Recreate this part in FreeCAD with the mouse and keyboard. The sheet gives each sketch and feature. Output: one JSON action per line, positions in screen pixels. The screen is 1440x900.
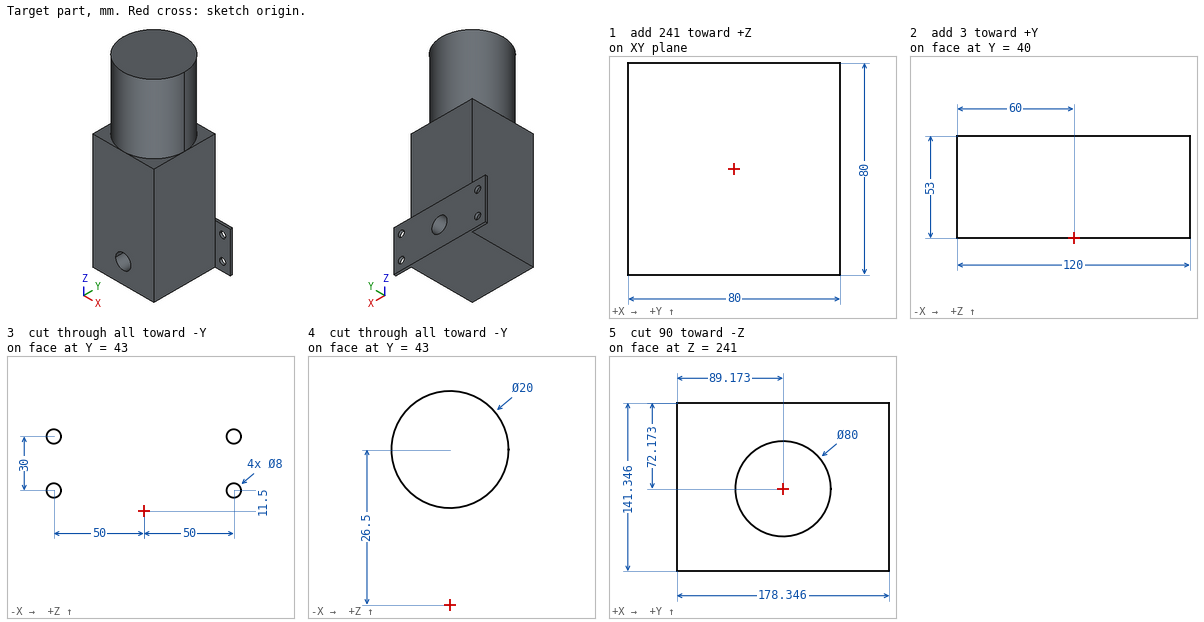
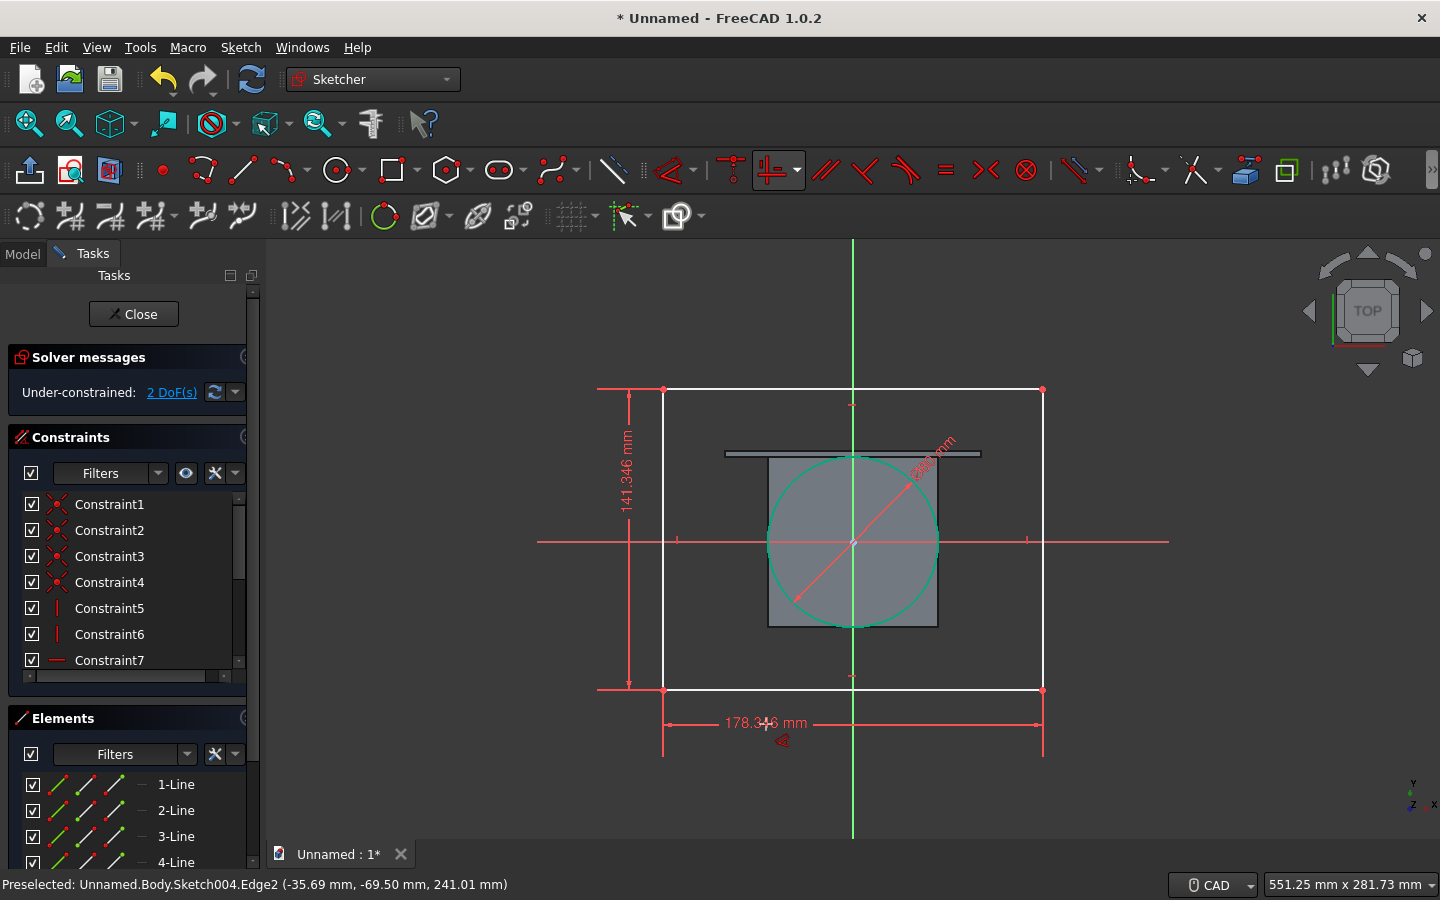
{"action": "left_click", "coordinate": [663, 389]}
{"action": "left_click", "coordinate": [758, 355]}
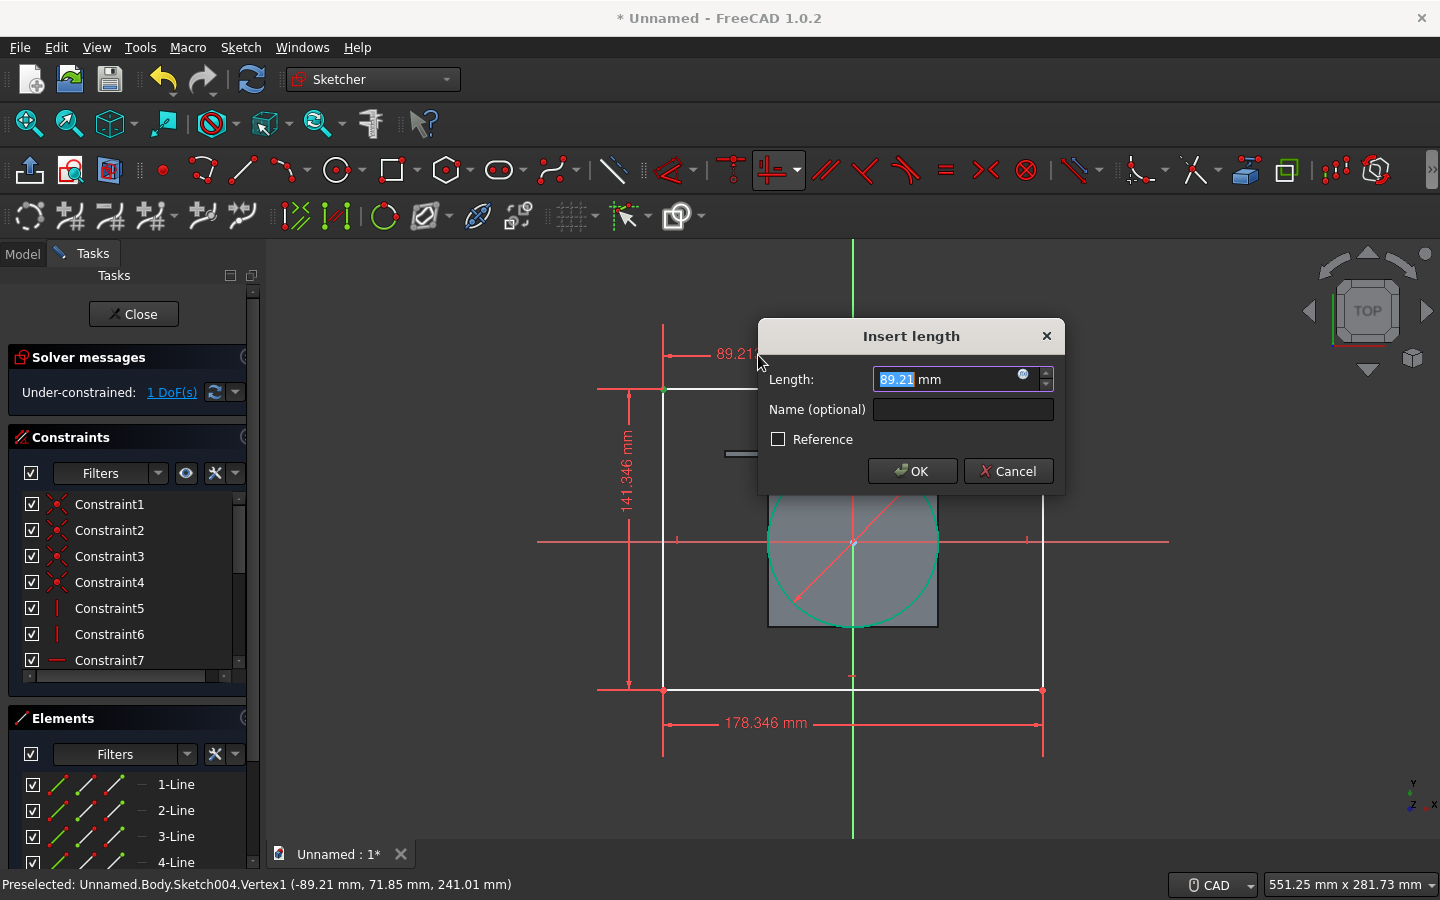
{"action": "type", "text": "89.173"}
{"action": "key", "text": "Return"}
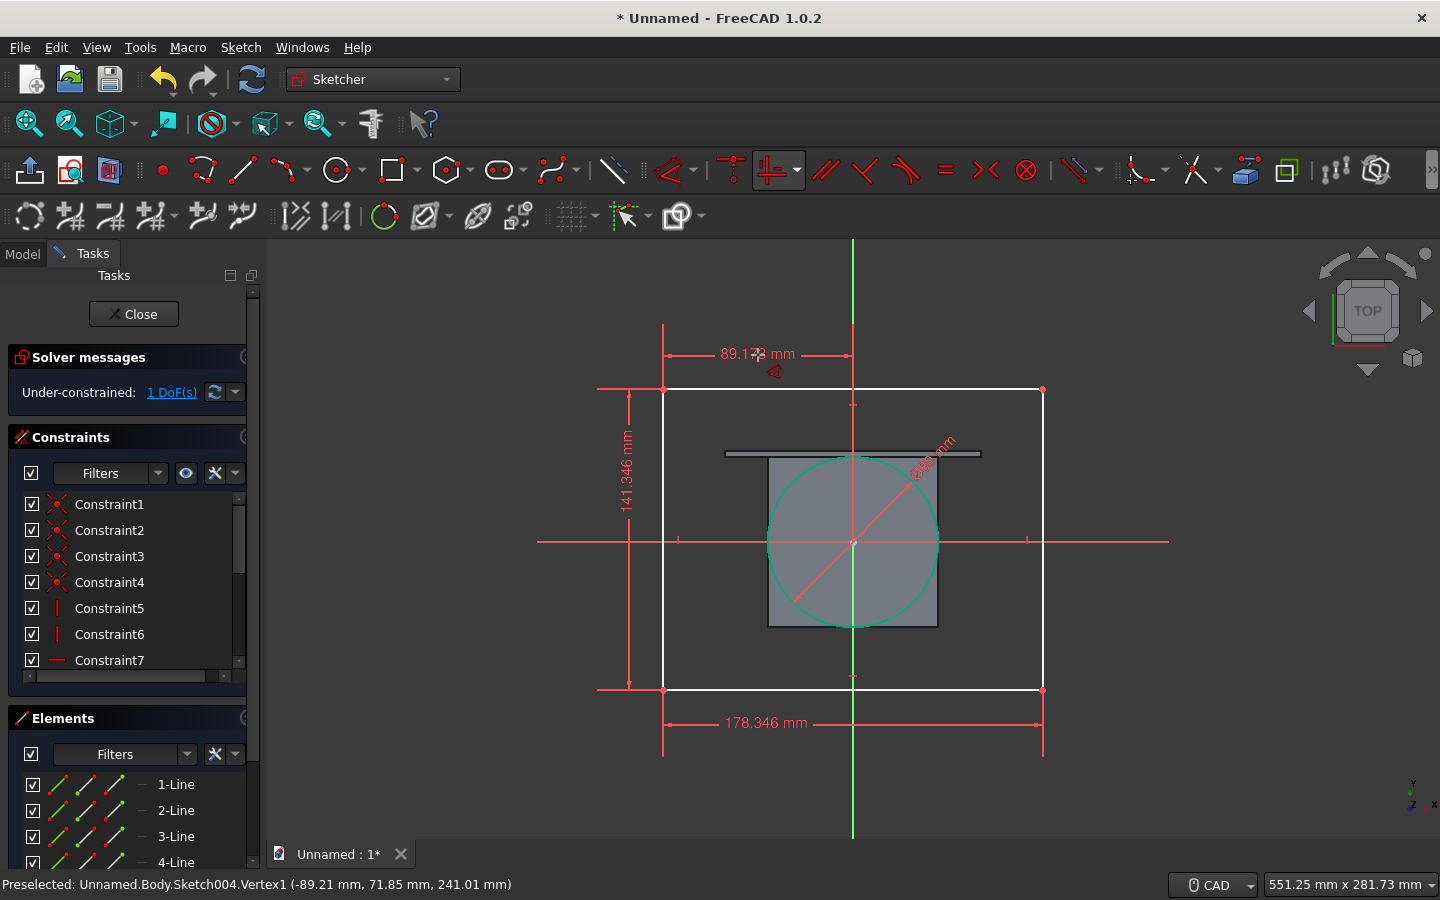
{"action": "left_click", "coordinate": [663, 389]}
{"action": "left_click", "coordinate": [629, 430]}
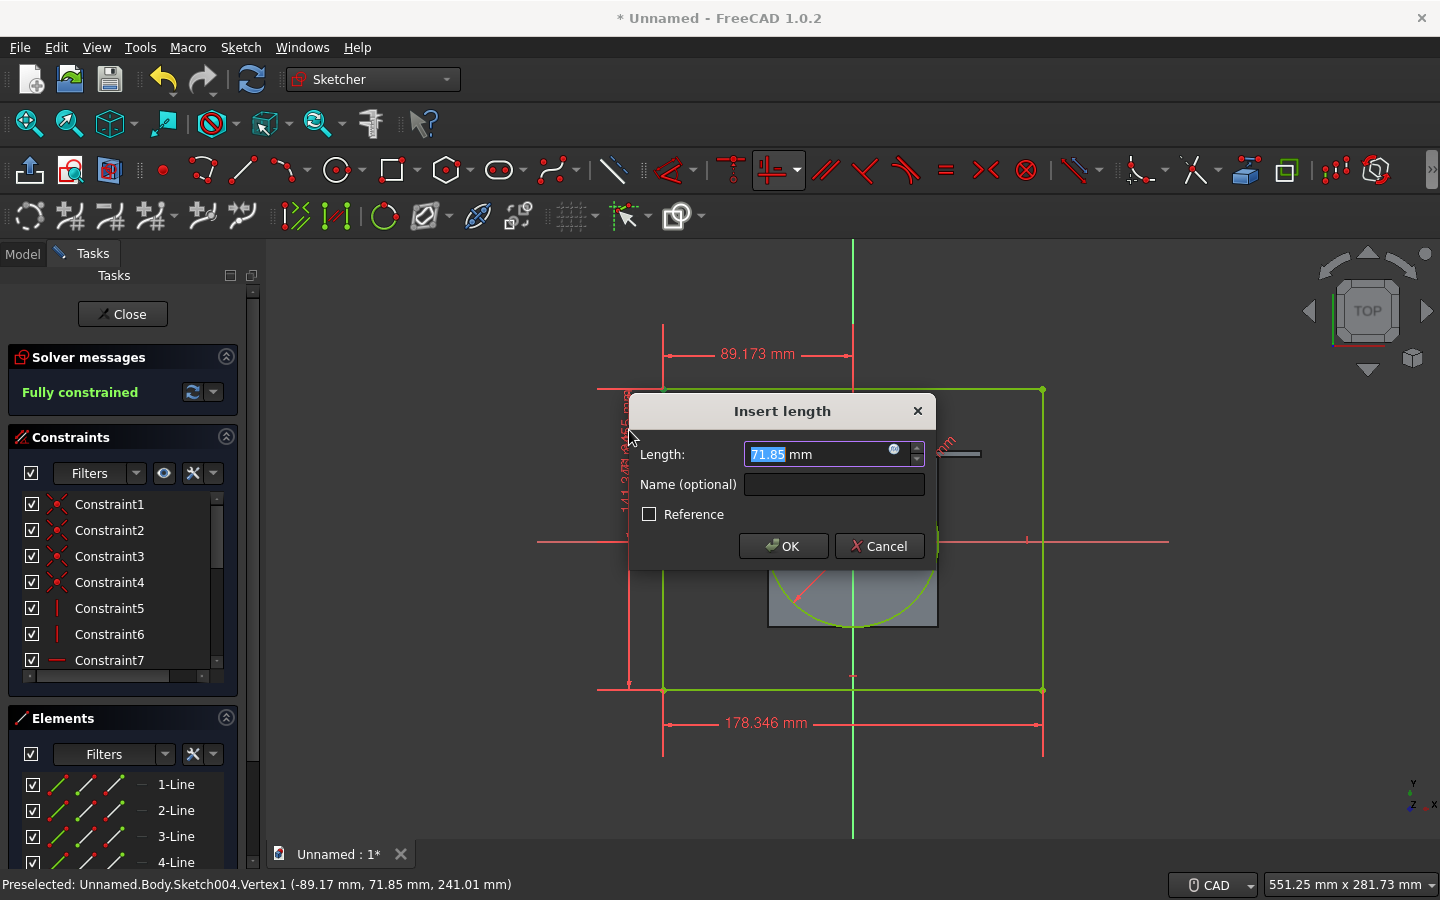
{"action": "type", "text": "72.173"}
{"action": "key", "text": "Return"}
{"action": "key", "text": "Escape"}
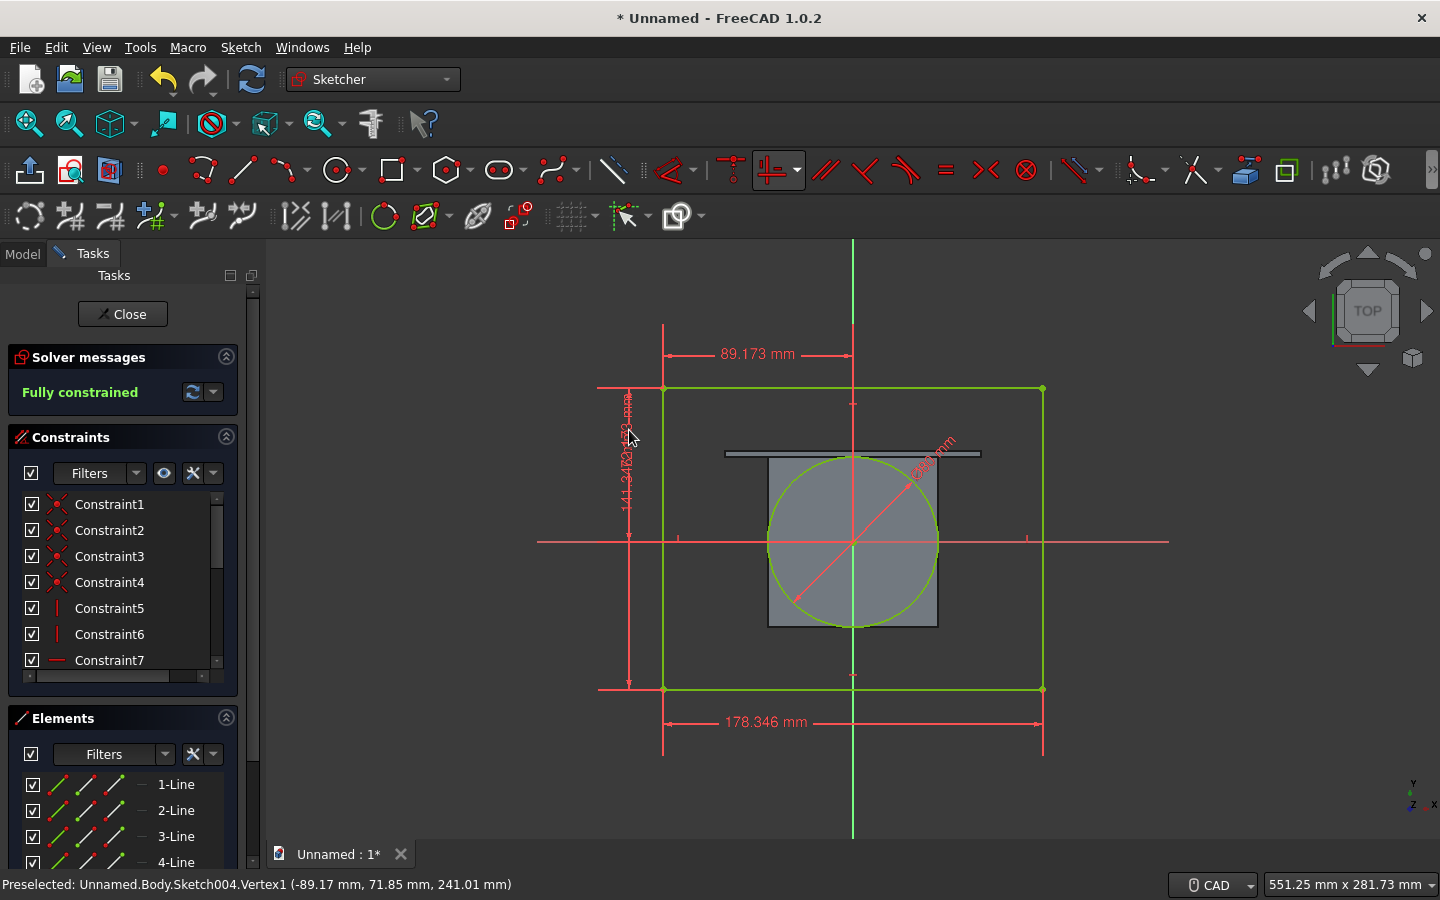
{"action": "left_click", "coordinate": [123, 314]}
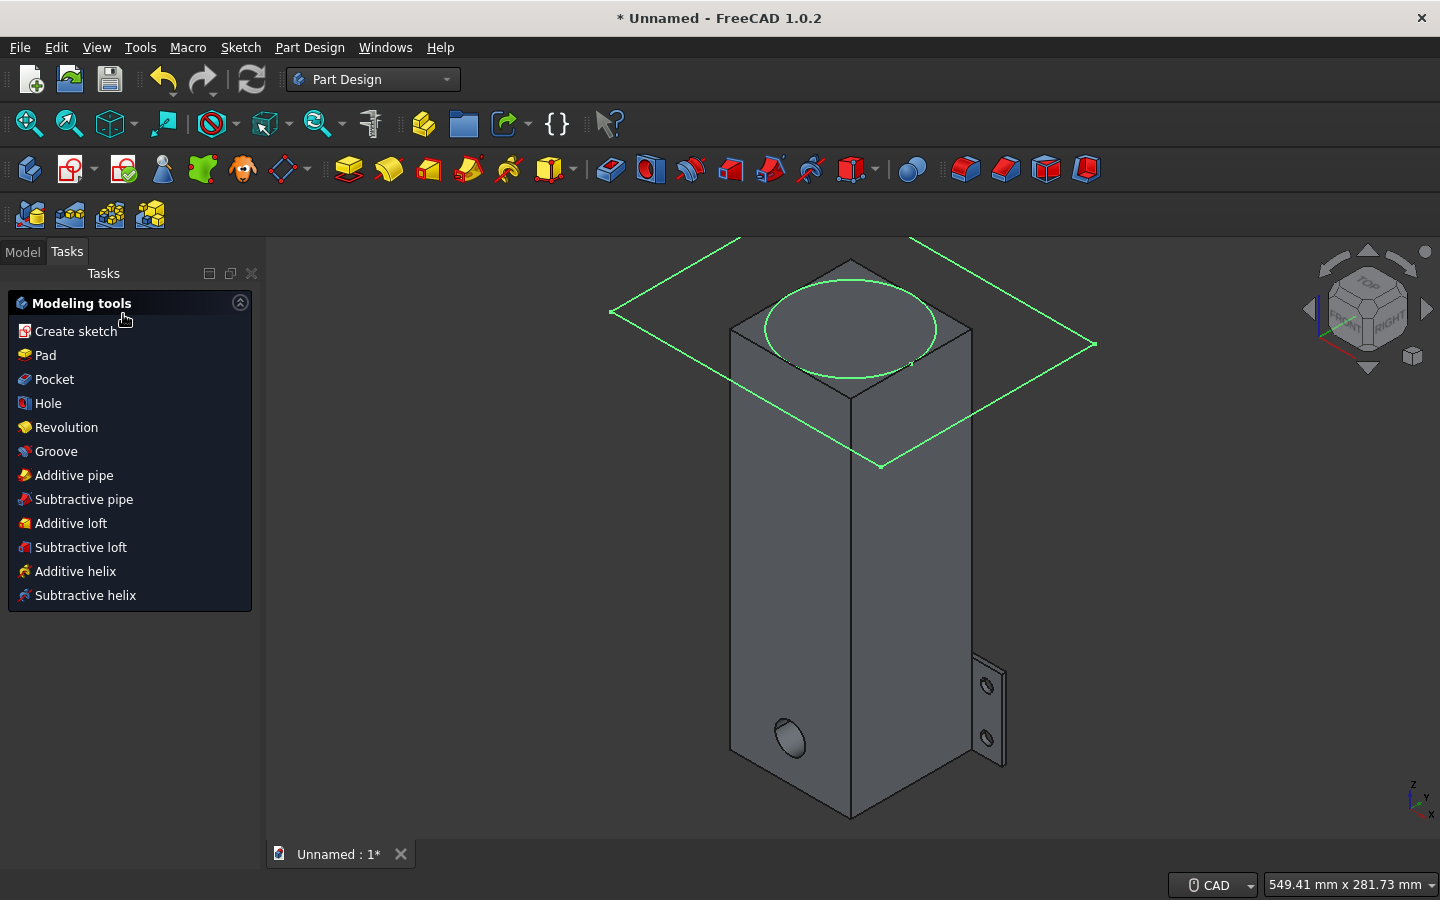
{"action": "left_click", "coordinate": [612, 170]}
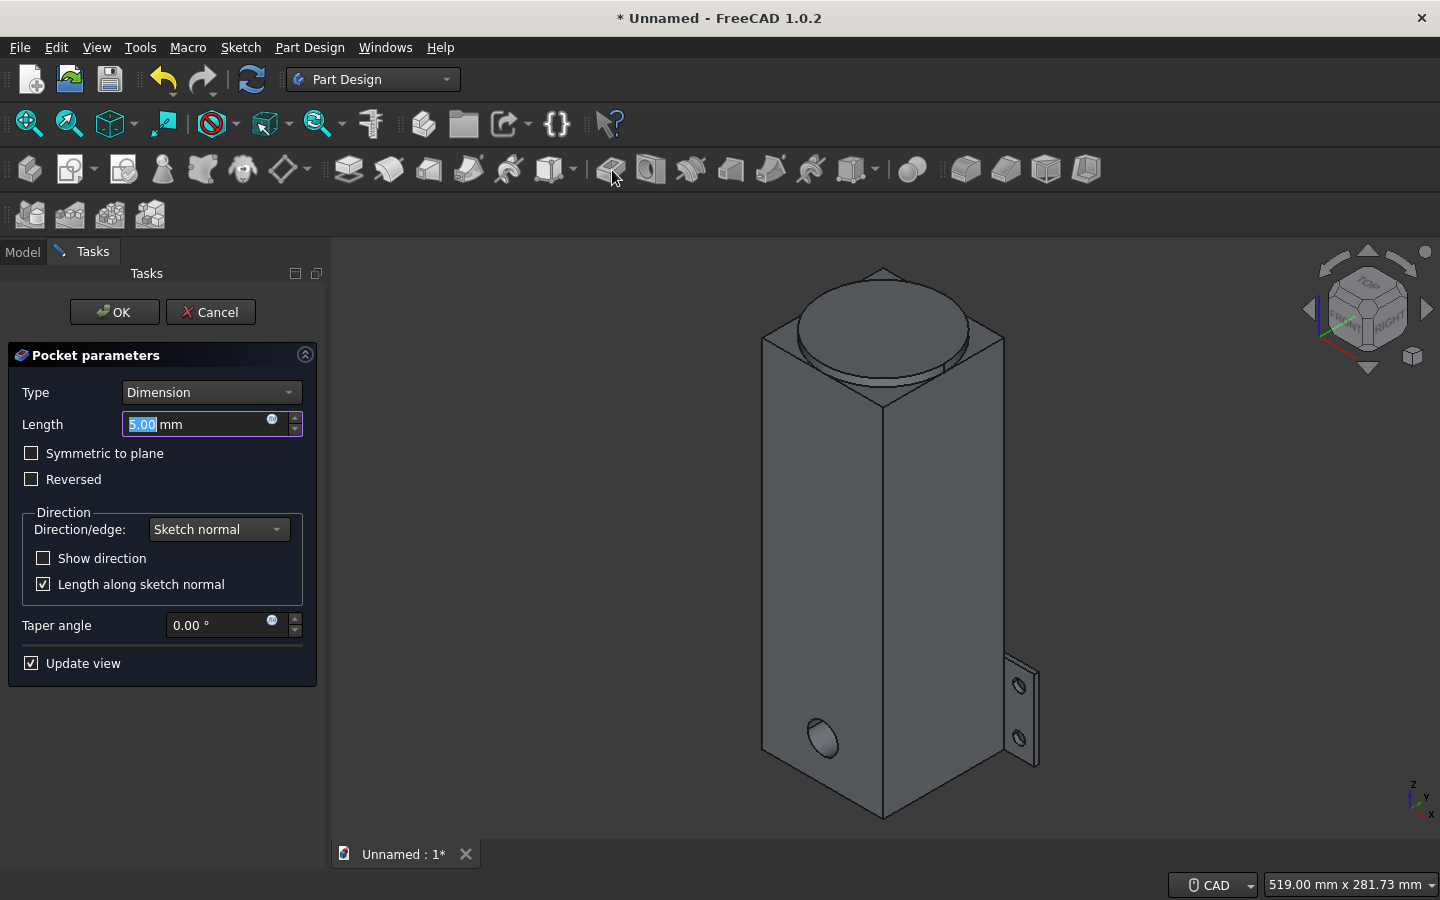
{"action": "type", "text": "90"}
{"action": "key", "text": "Tab"}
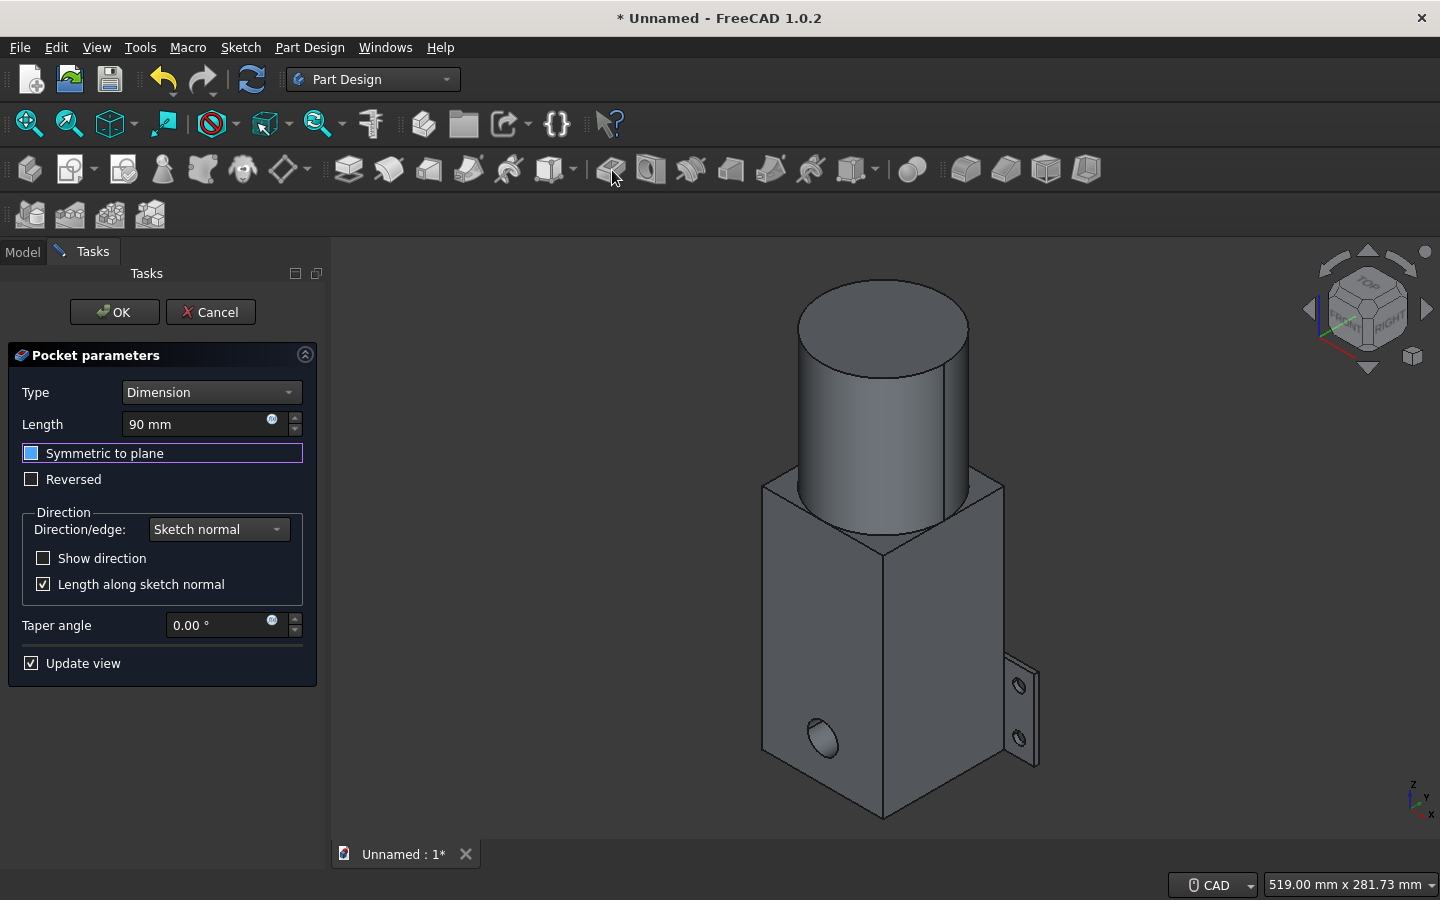
{"action": "left_click", "coordinate": [115, 312]}